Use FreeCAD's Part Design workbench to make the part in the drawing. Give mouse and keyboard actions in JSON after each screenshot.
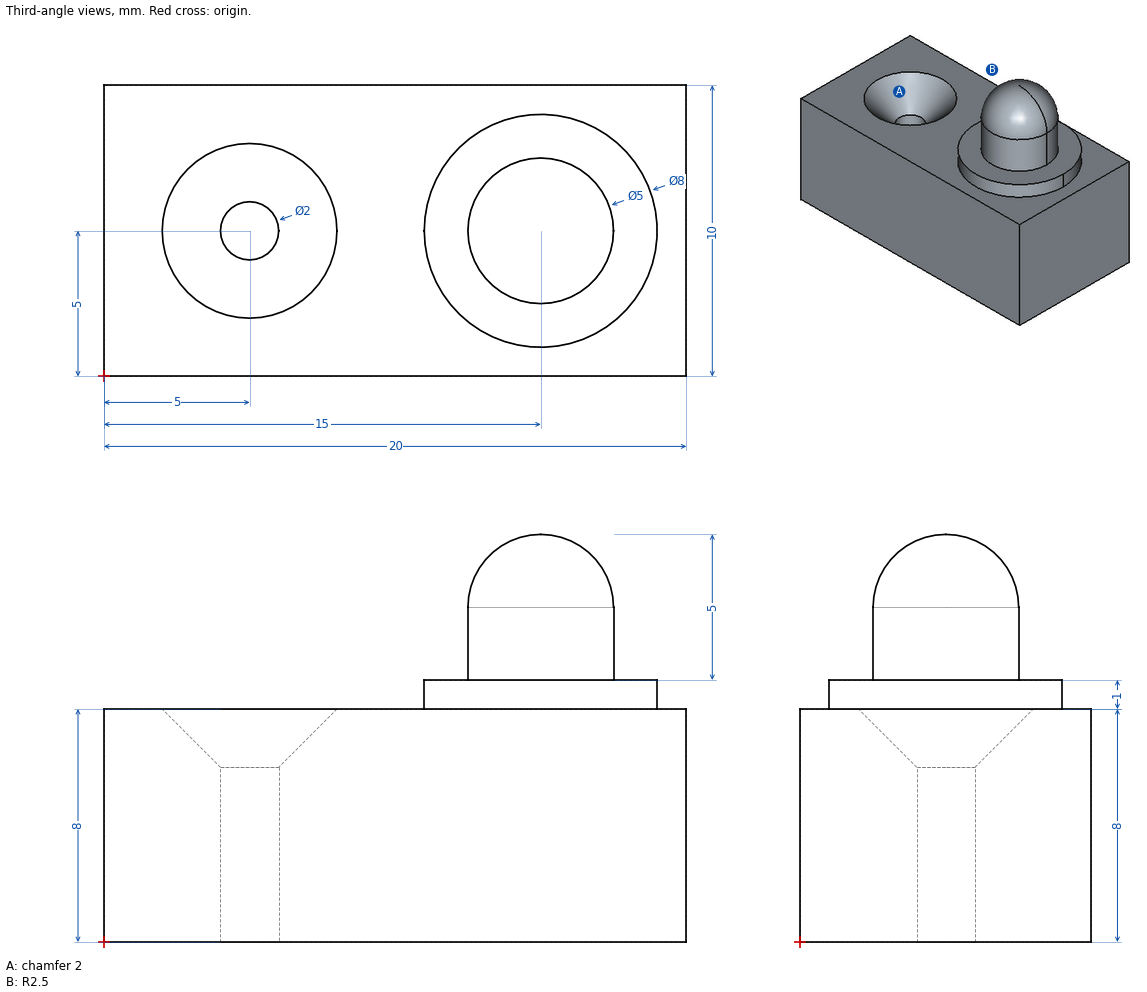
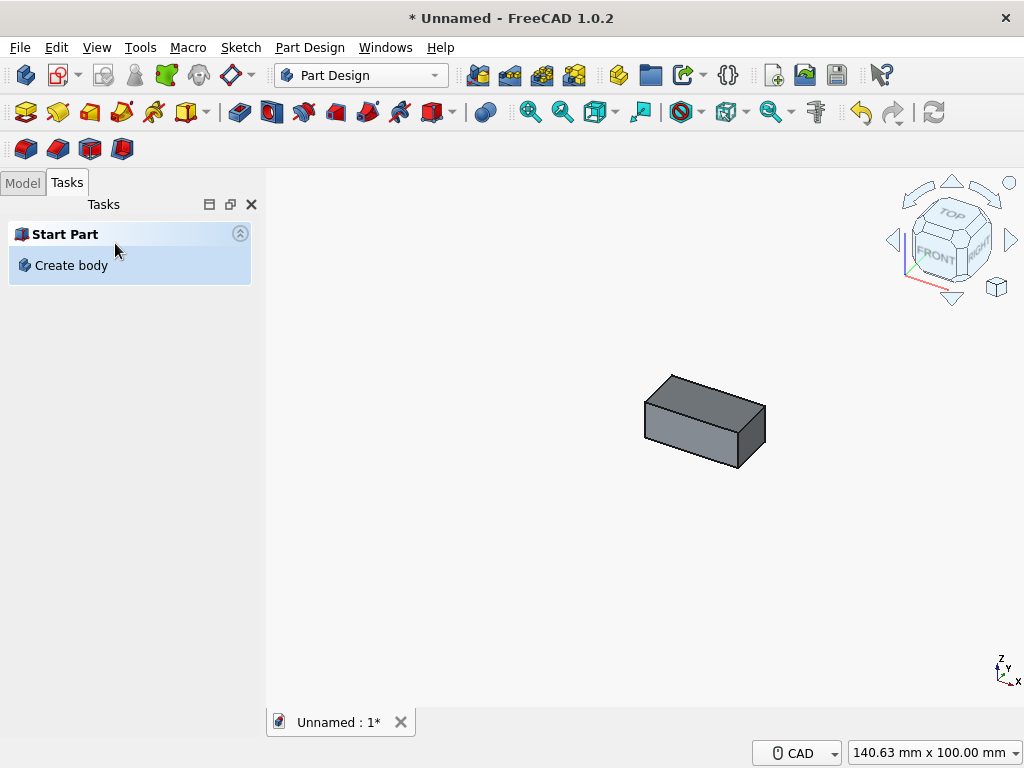
{"action": "left_click", "coordinate": [532, 112]}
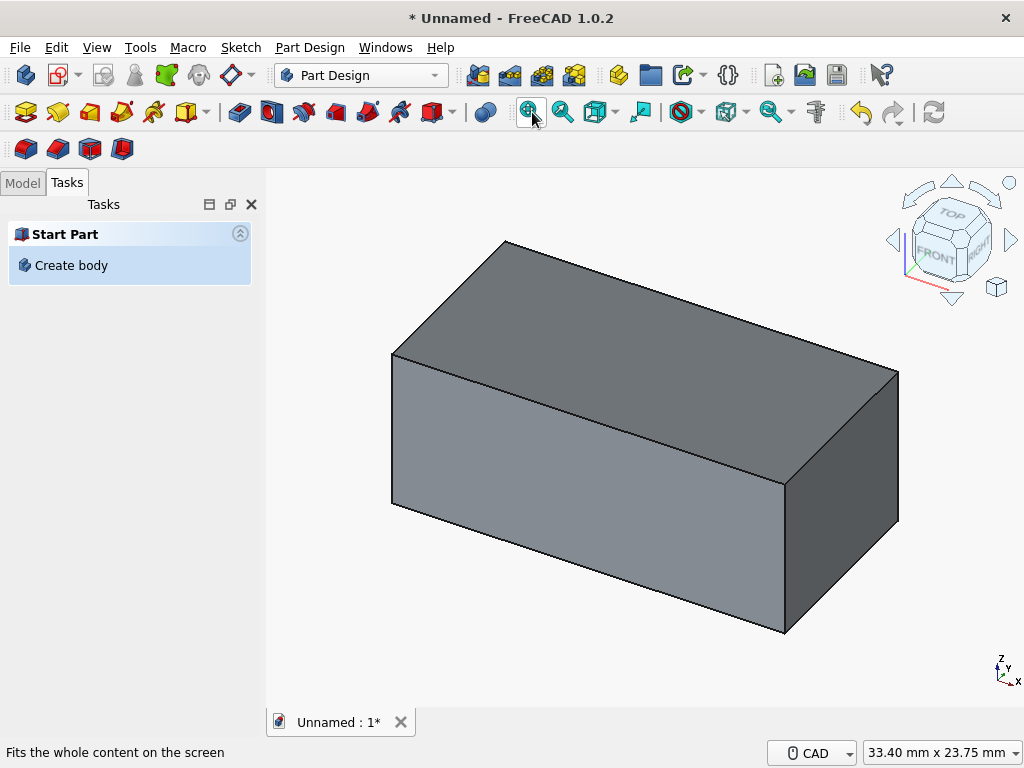
{"action": "left_click", "coordinate": [701, 381]}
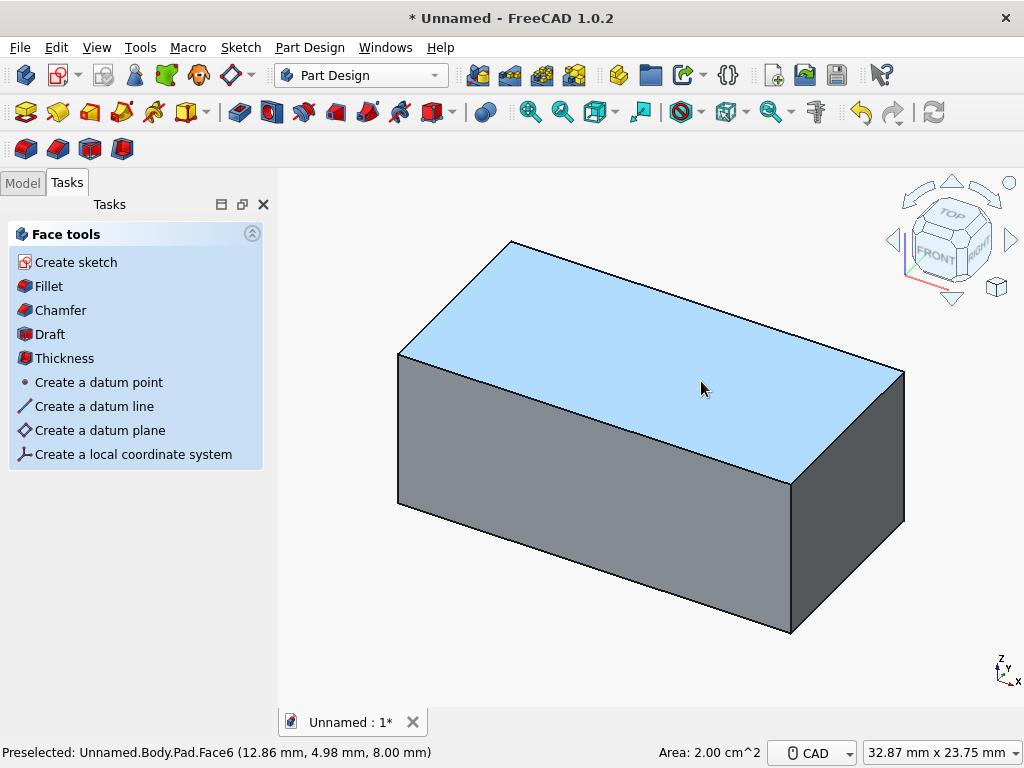
{"action": "left_click", "coordinate": [58, 76]}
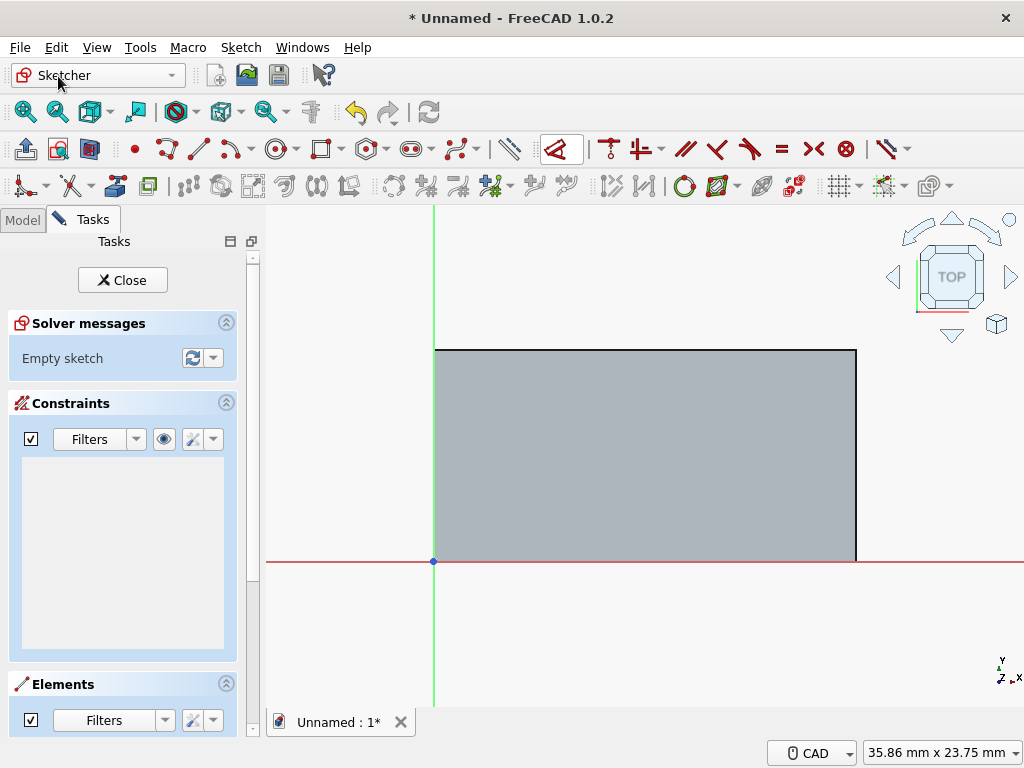
{"action": "scroll", "coordinate": [533, 456], "scroll_direction": "up", "scroll_amount": 10}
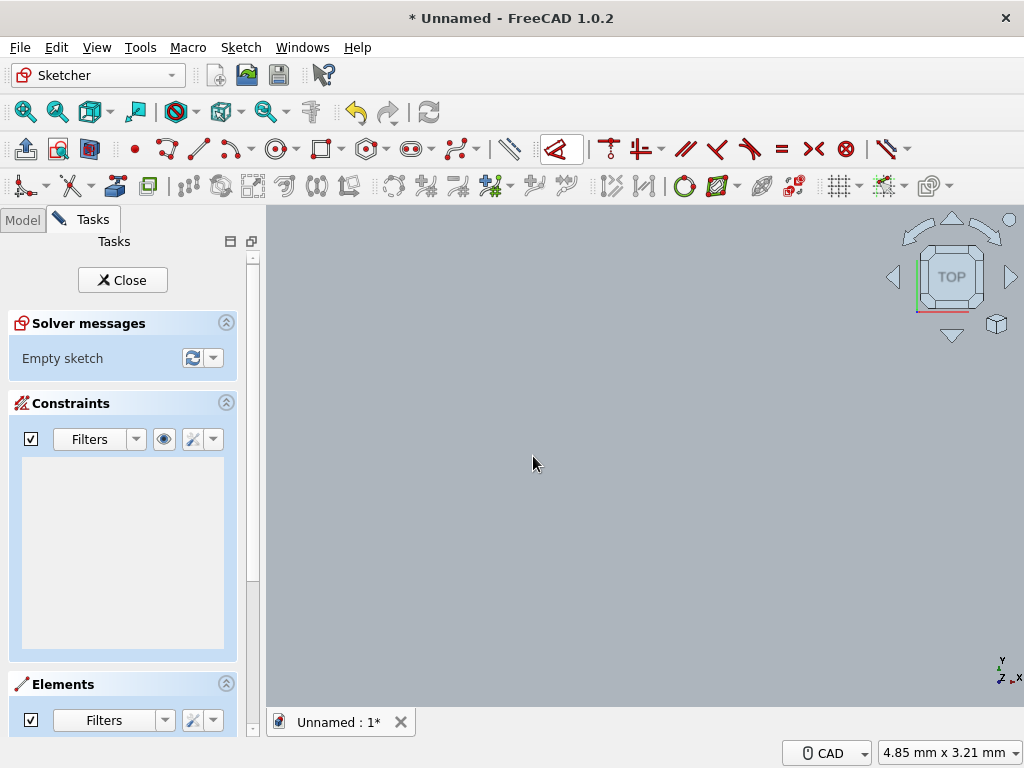
{"action": "left_click", "coordinate": [276, 150]}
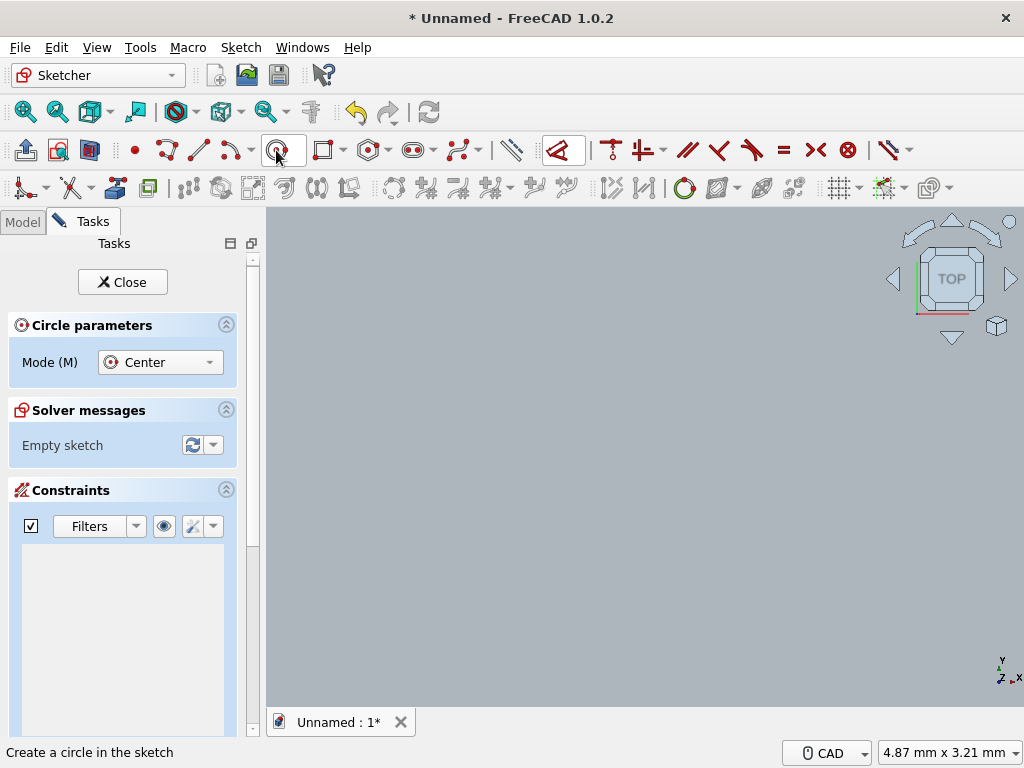
{"action": "left_click", "coordinate": [578, 454]}
{"action": "mouse_move", "coordinate": [688, 344]}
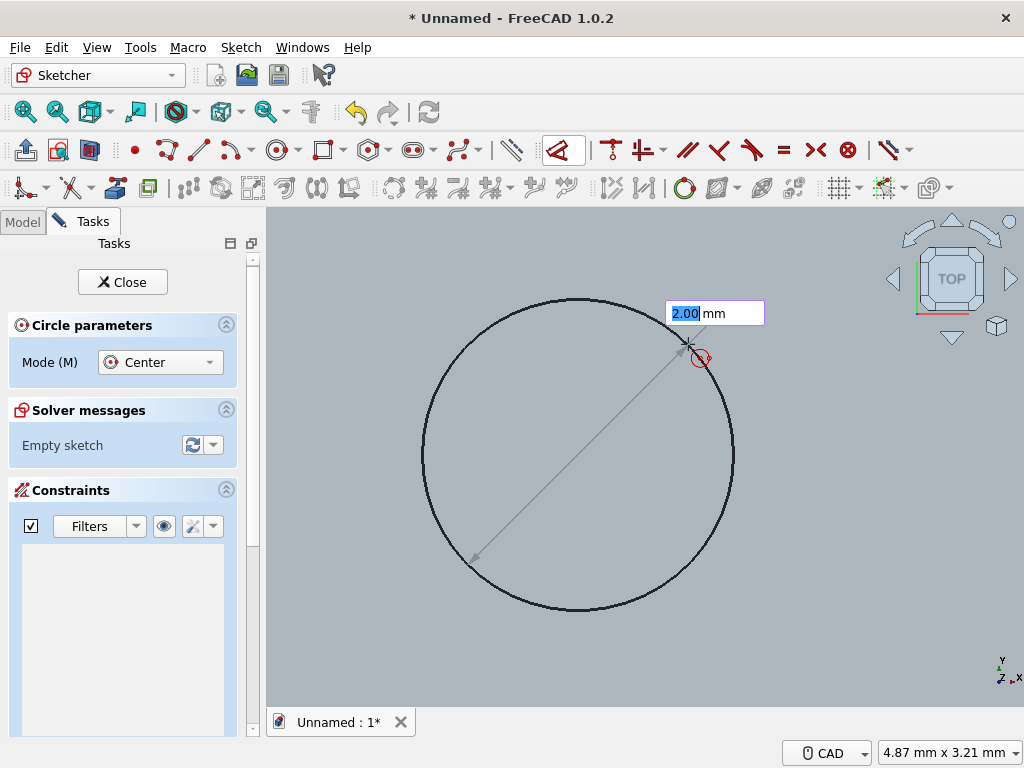
{"action": "type", "text": "2"}
{"action": "key", "text": "Return"}
{"action": "key", "text": "Escape"}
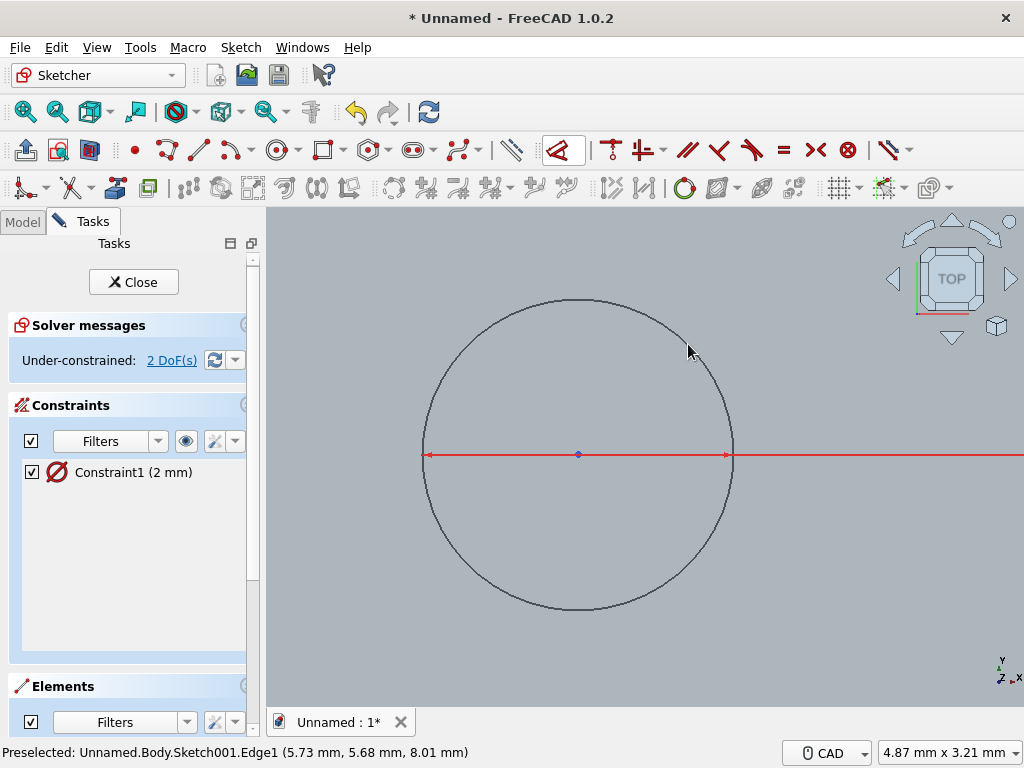
{"action": "left_click", "coordinate": [558, 150]}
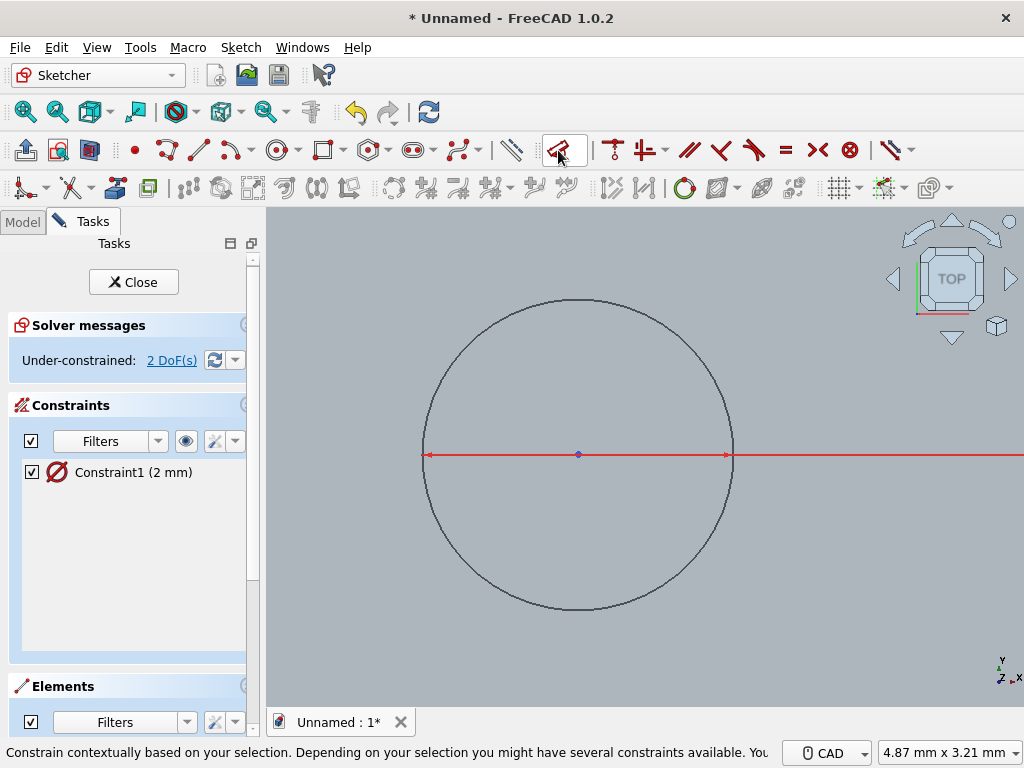
{"action": "left_click", "coordinate": [578, 455]}
{"action": "left_click", "coordinate": [371, 421]}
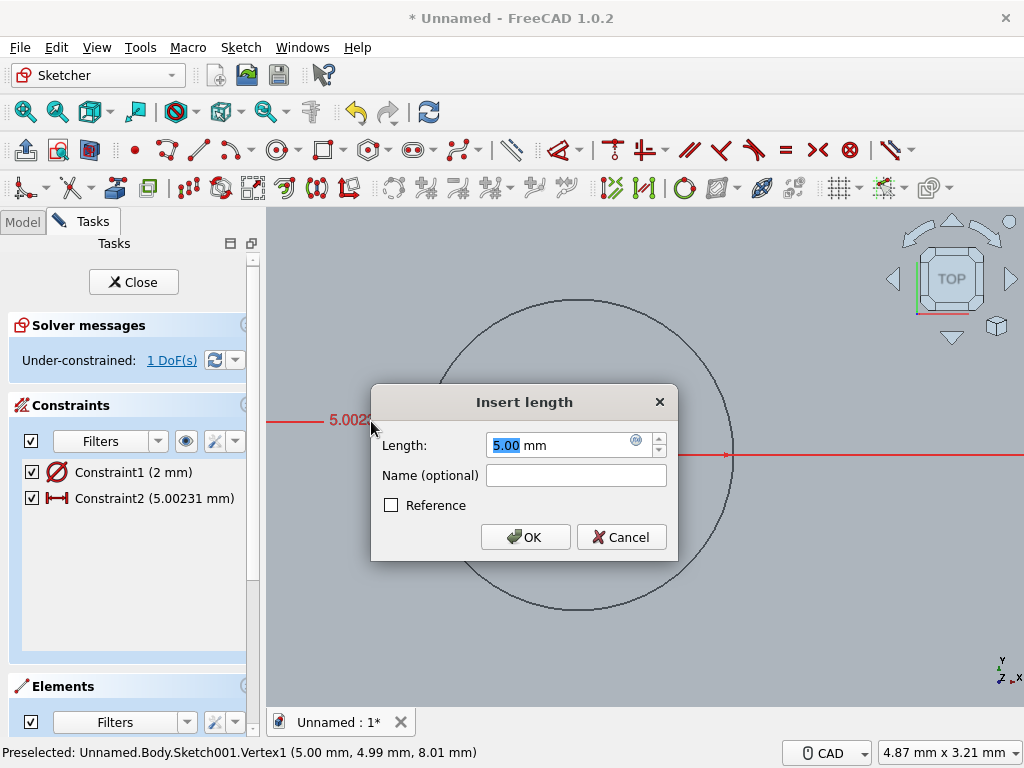
{"action": "type", "text": "5"}
{"action": "key", "text": "Return"}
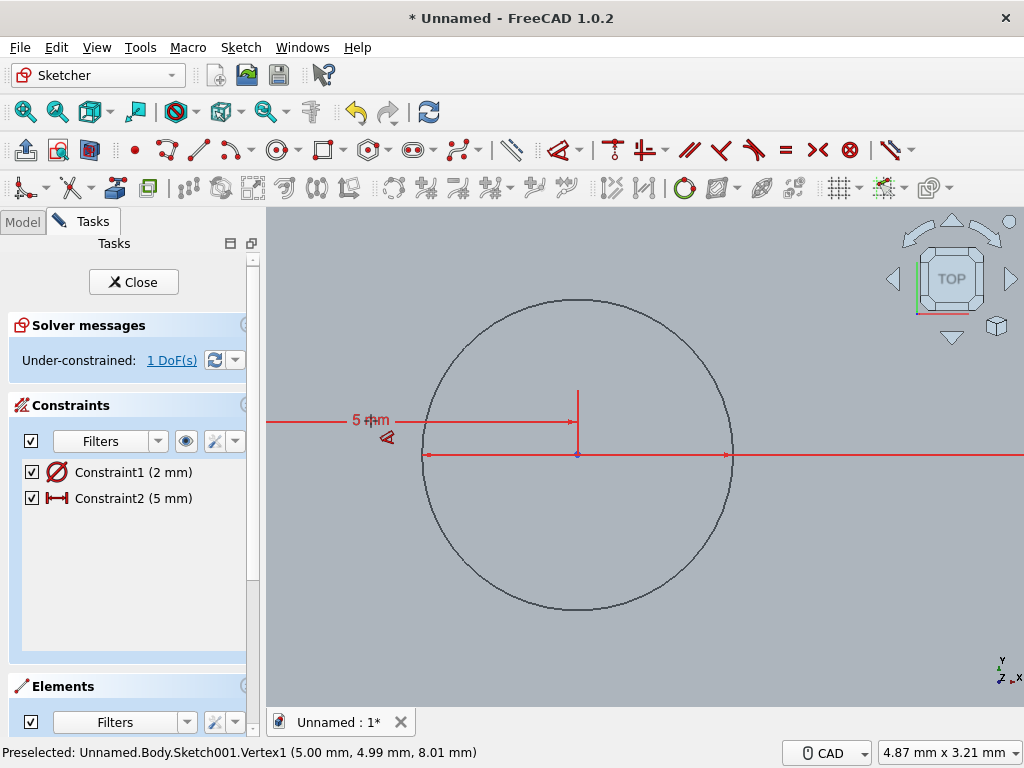
{"action": "left_click", "coordinate": [578, 455]}
{"action": "left_click", "coordinate": [612, 567]}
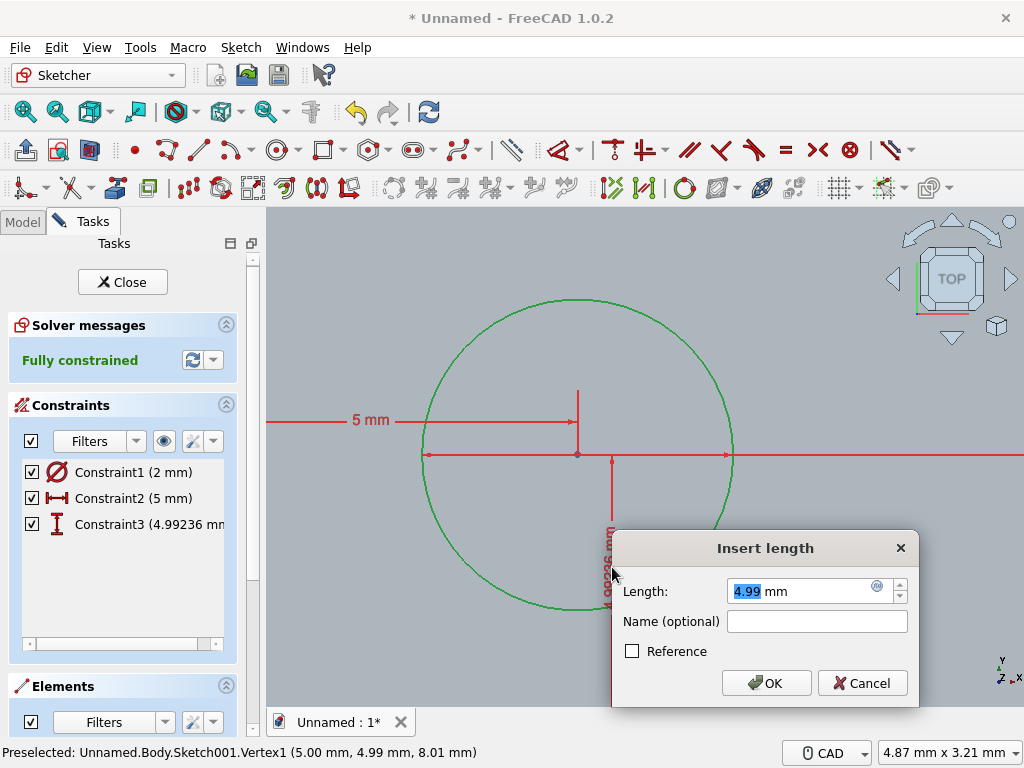
{"action": "type", "text": "5"}
{"action": "key", "text": "Return"}
{"action": "key", "text": "Escape"}